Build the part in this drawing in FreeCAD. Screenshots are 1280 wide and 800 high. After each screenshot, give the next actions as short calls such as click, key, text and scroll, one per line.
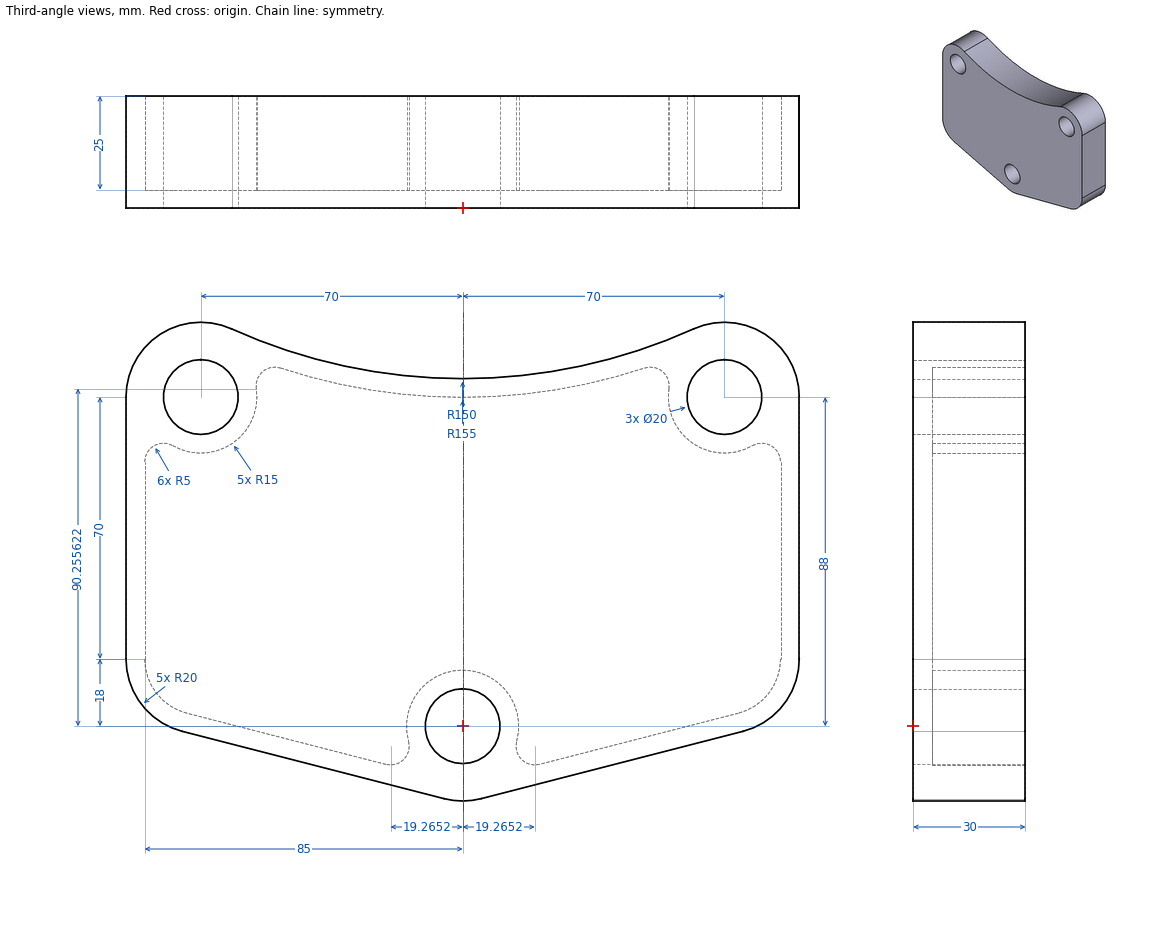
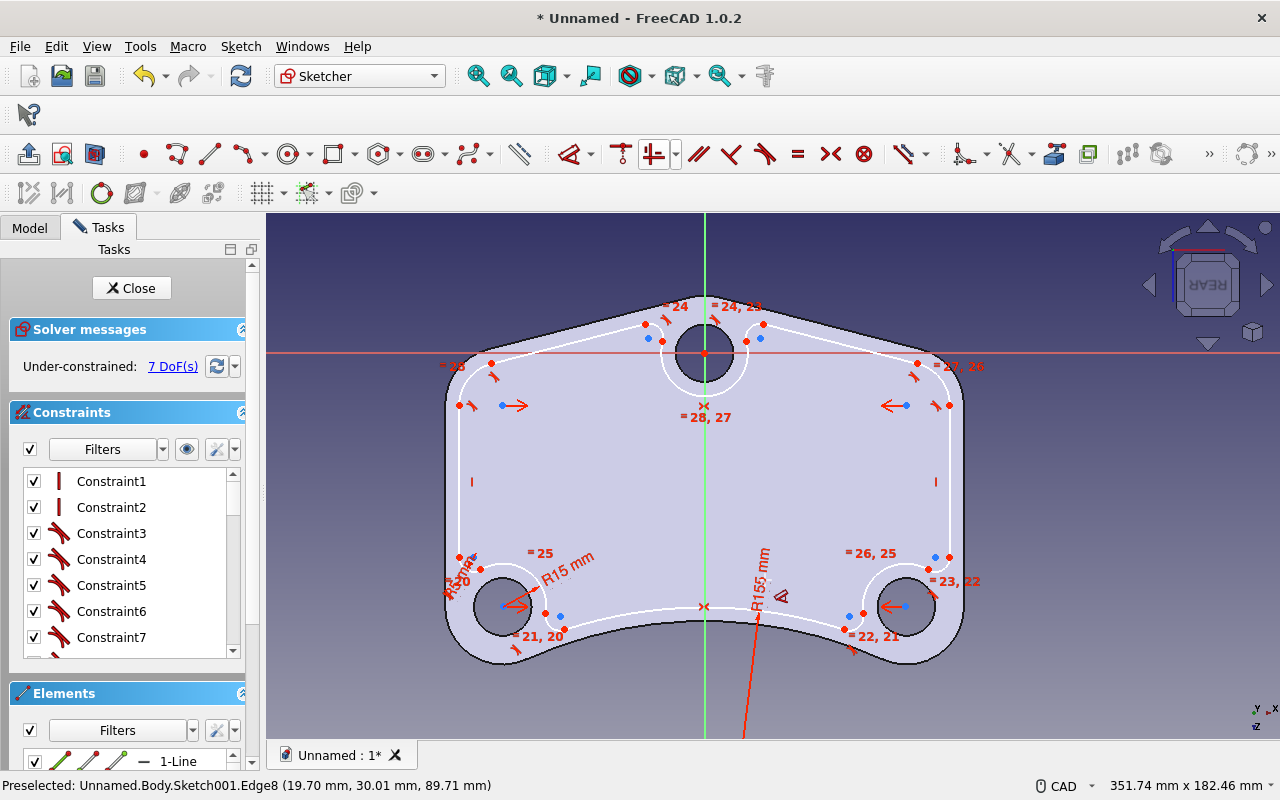
click(459, 406)
click(582, 319)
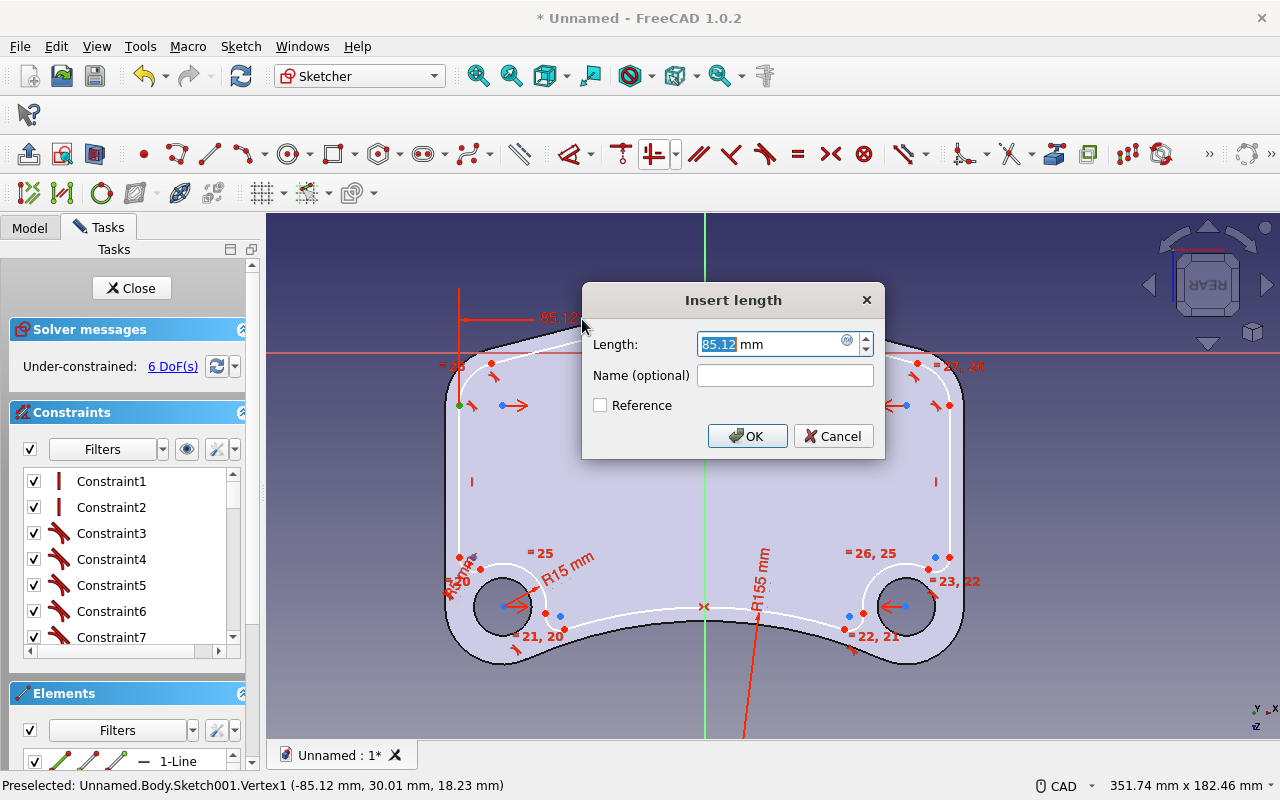
text(85)
key(Return)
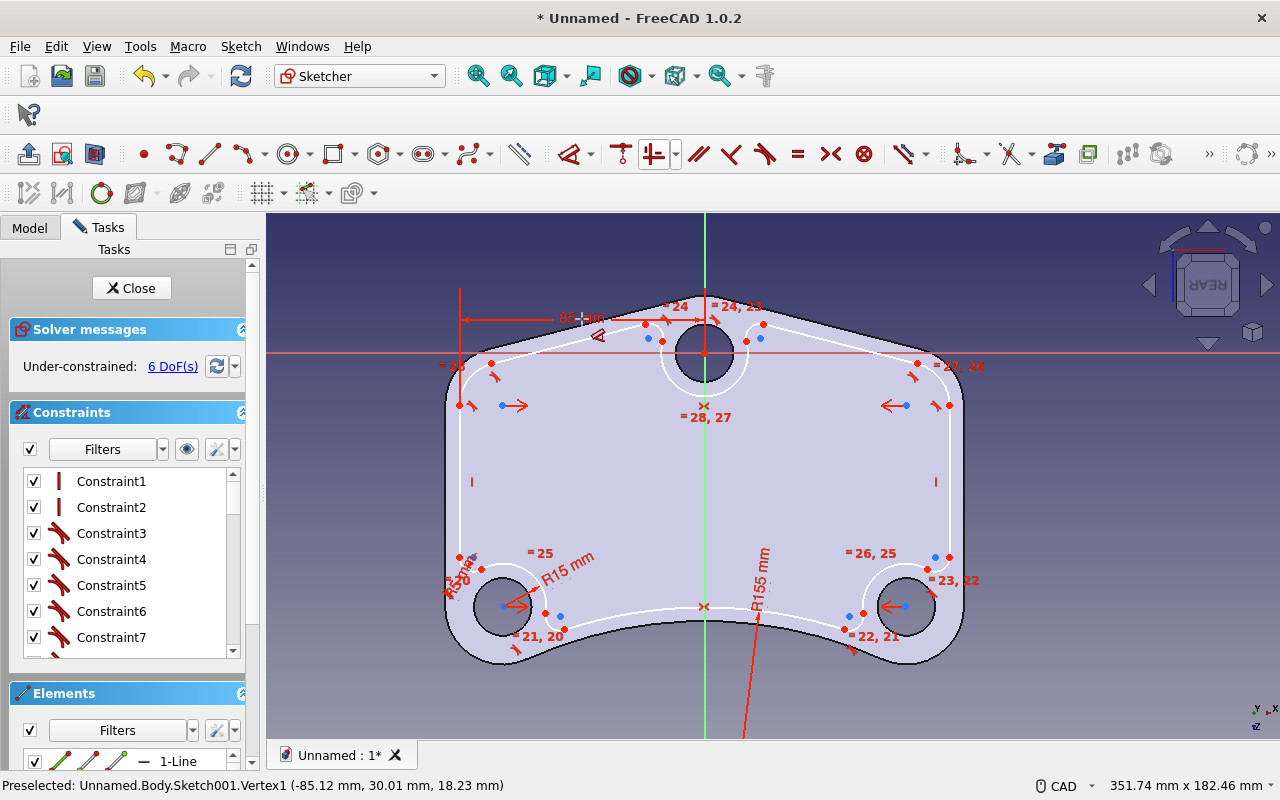
click(460, 406)
click(426, 379)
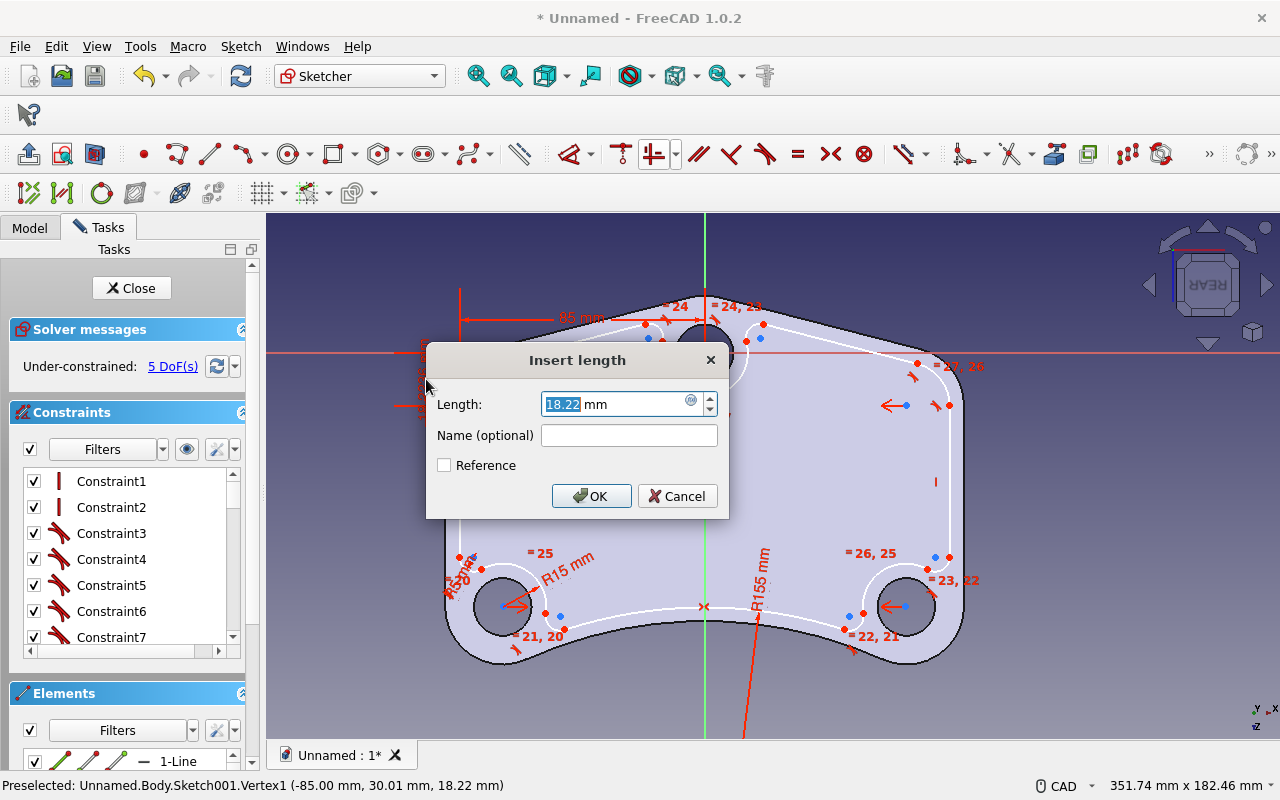
text(18)
key(Return)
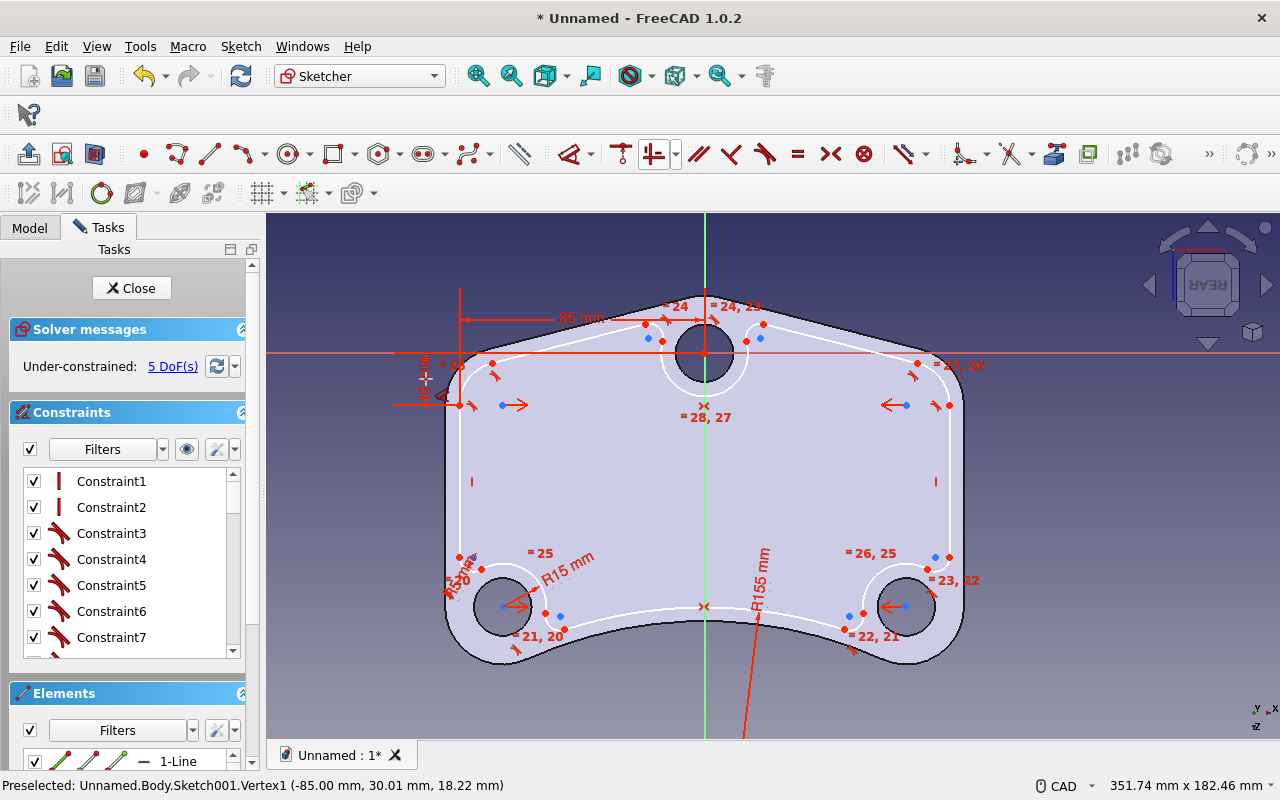
click(503, 607)
click(604, 641)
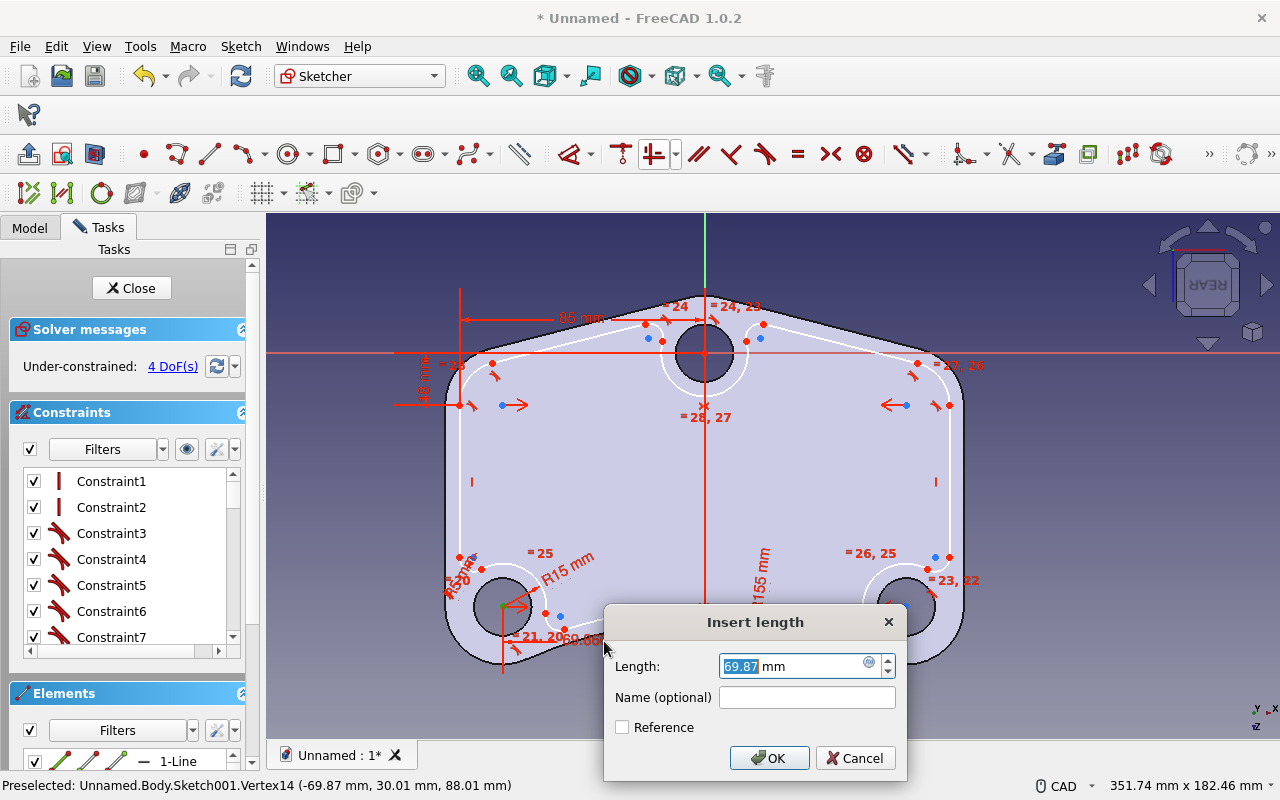
text(70)
key(Return)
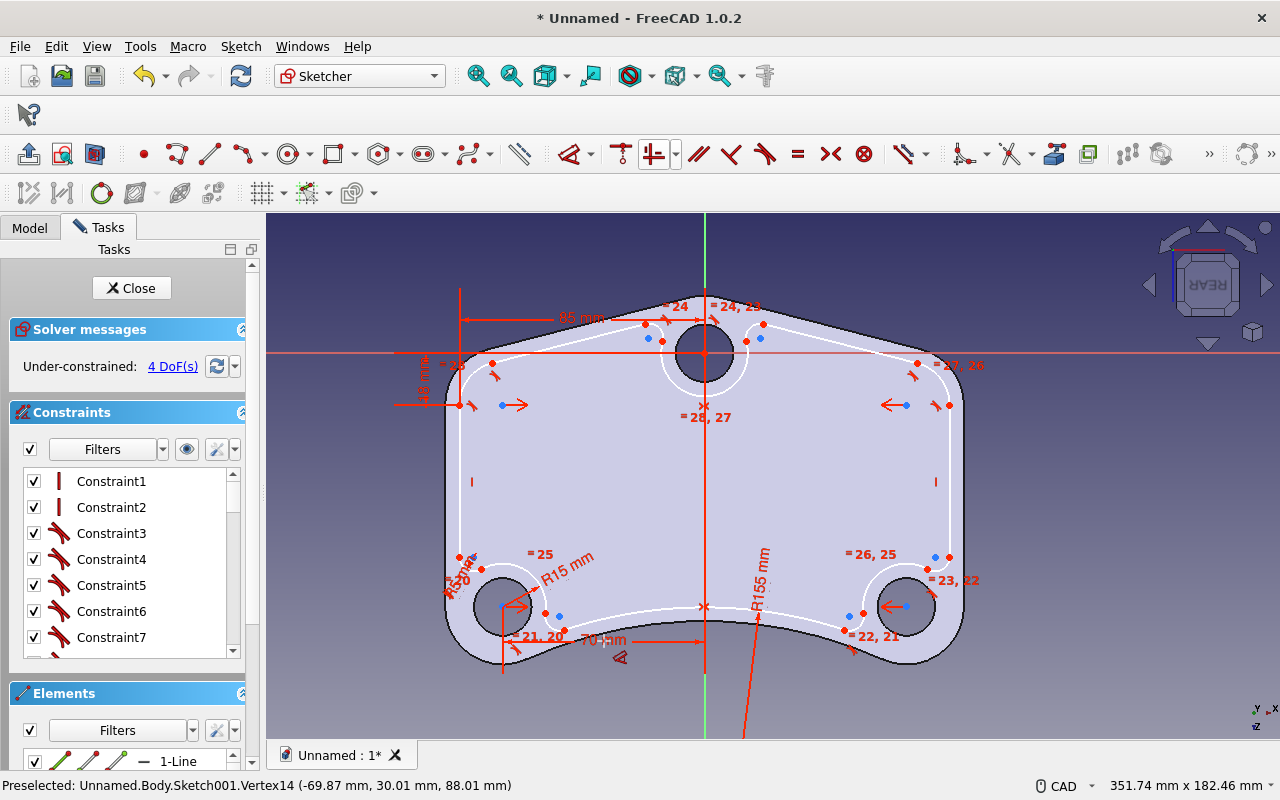
click(503, 607)
click(739, 480)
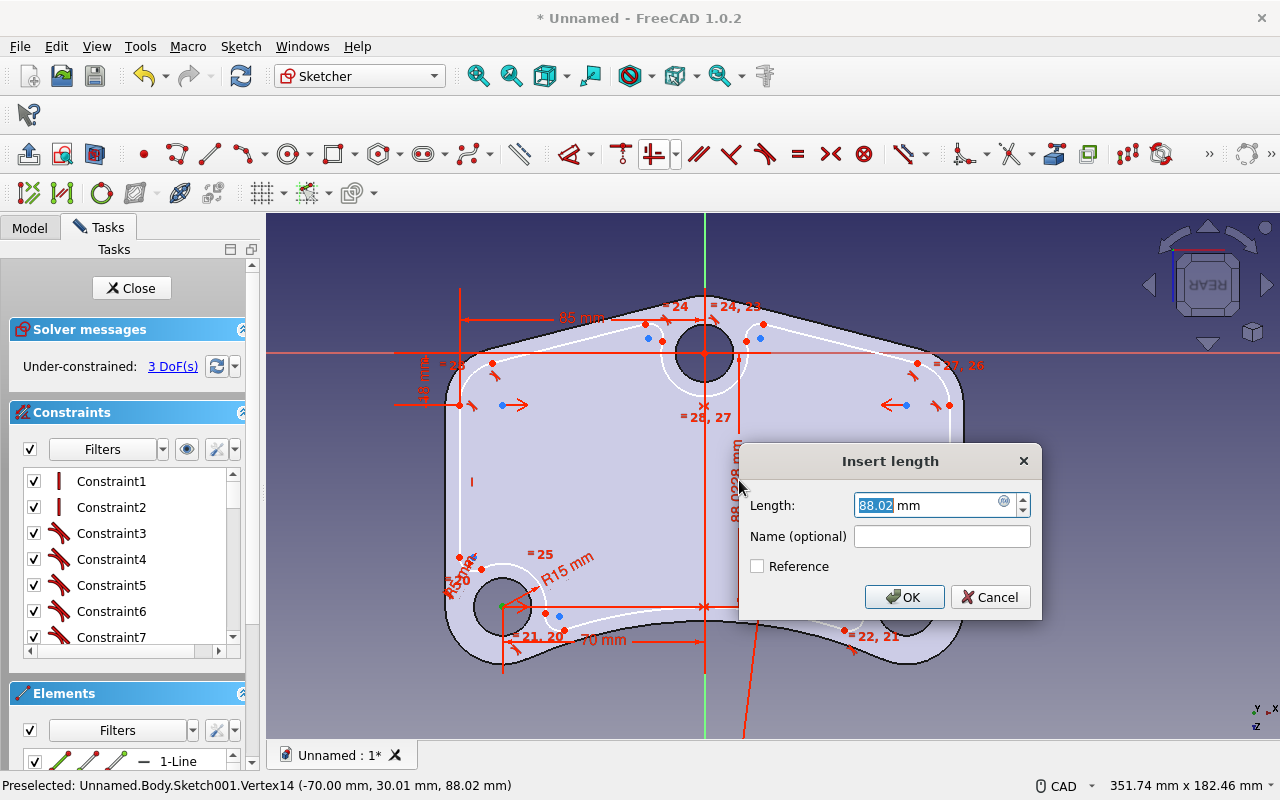
text(88)
key(Return)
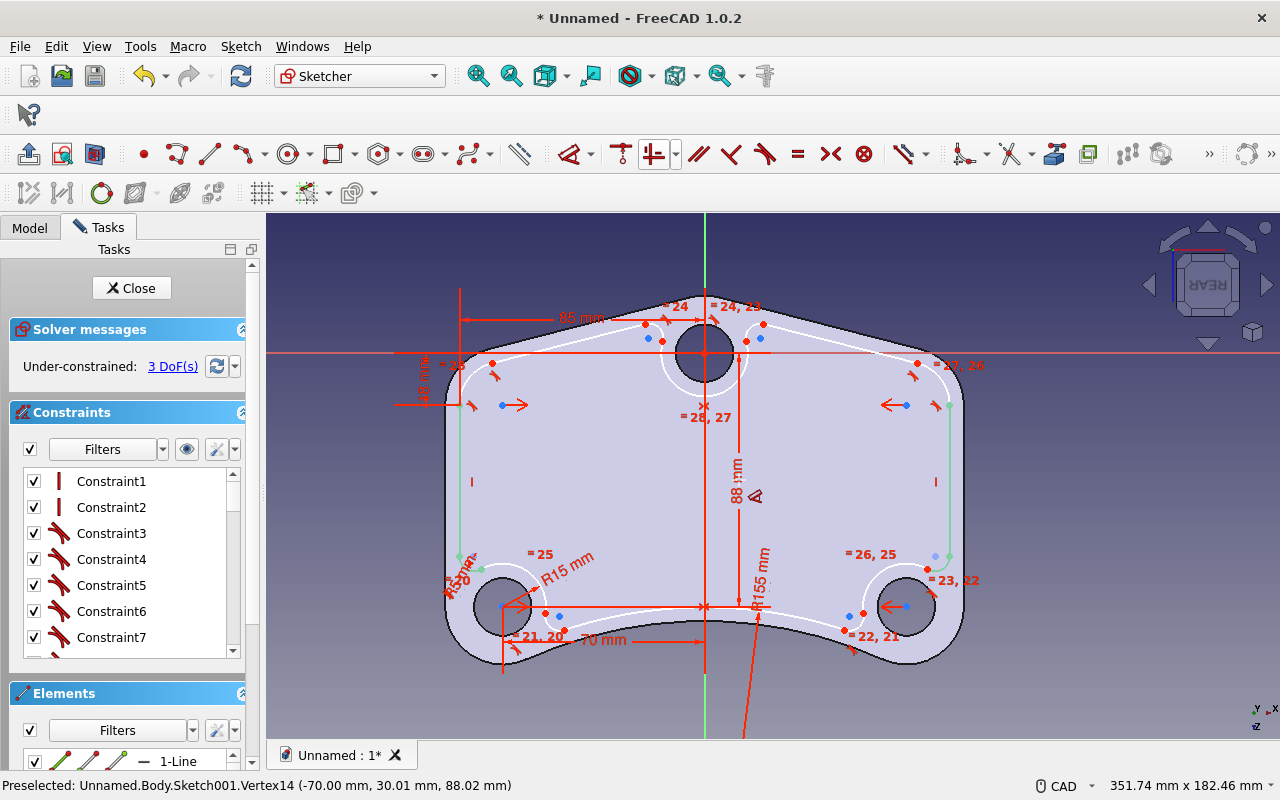
click(760, 338)
click(732, 304)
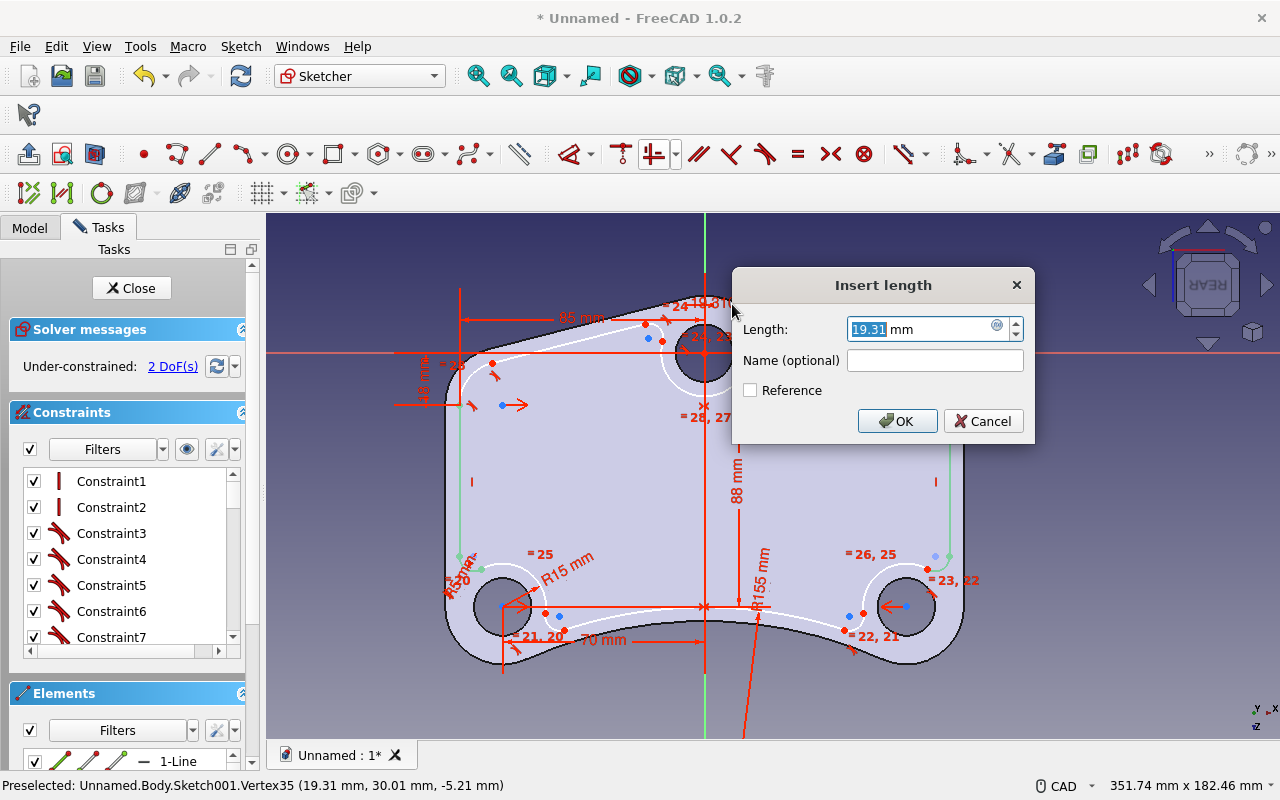
text(19.2652)
key(Return)